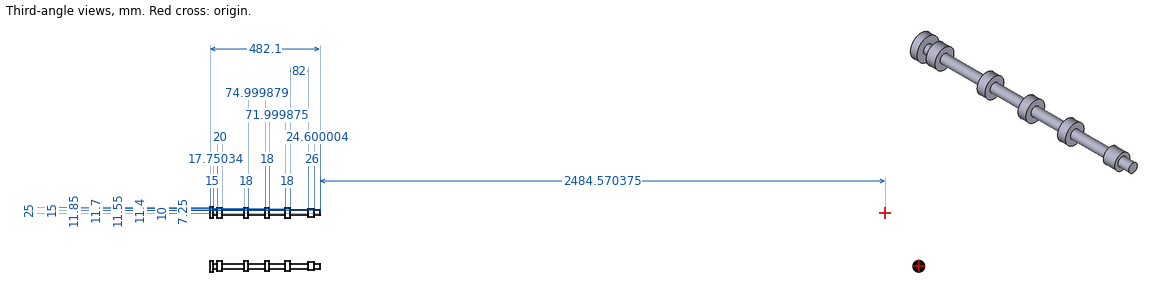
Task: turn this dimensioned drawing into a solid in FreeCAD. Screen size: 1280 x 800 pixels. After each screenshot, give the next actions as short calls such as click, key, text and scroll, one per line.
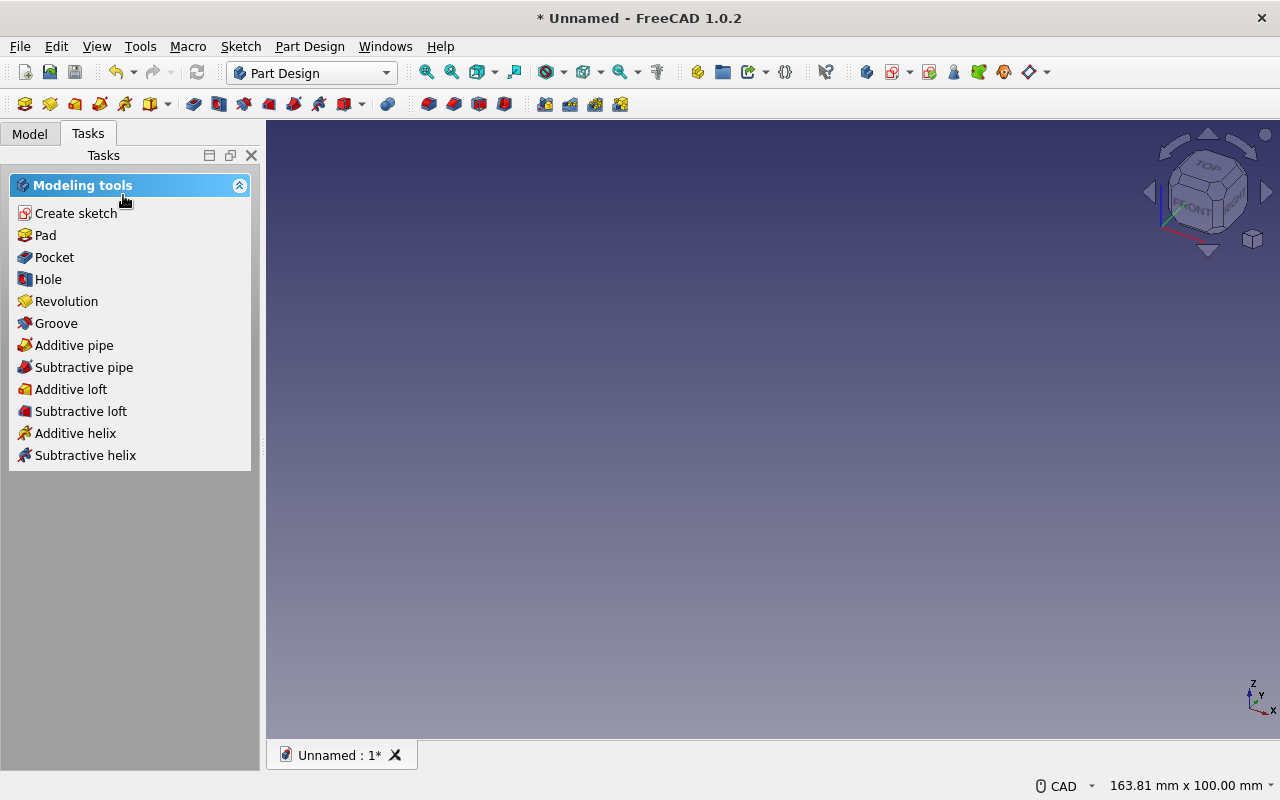
click(50, 104)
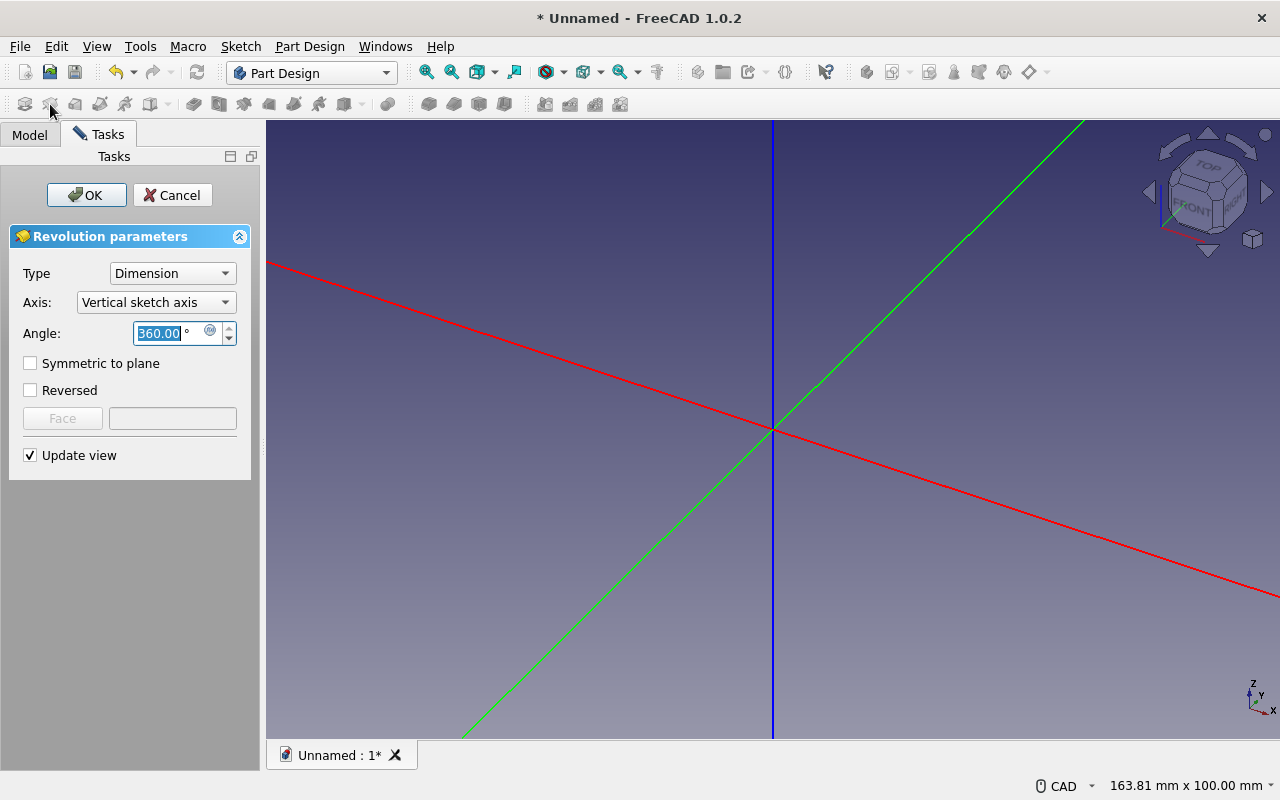
click(157, 302)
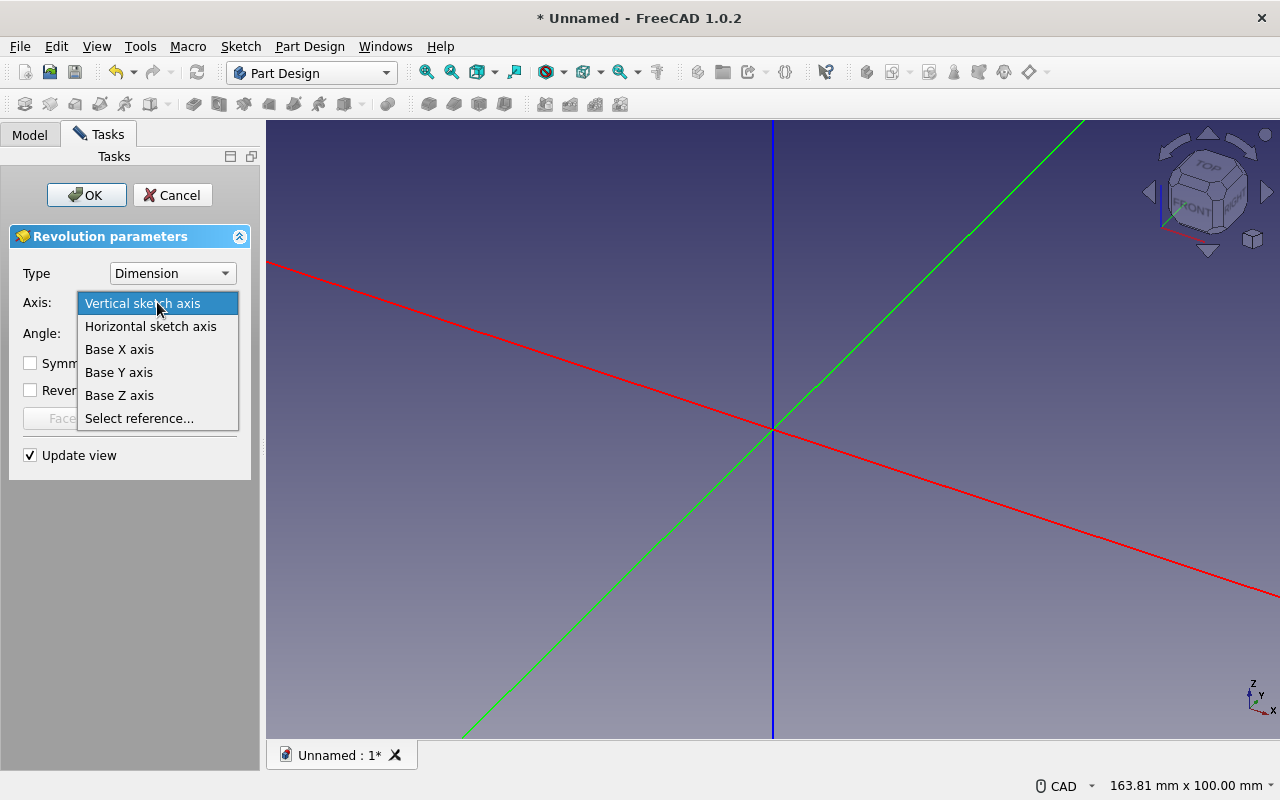
click(156, 326)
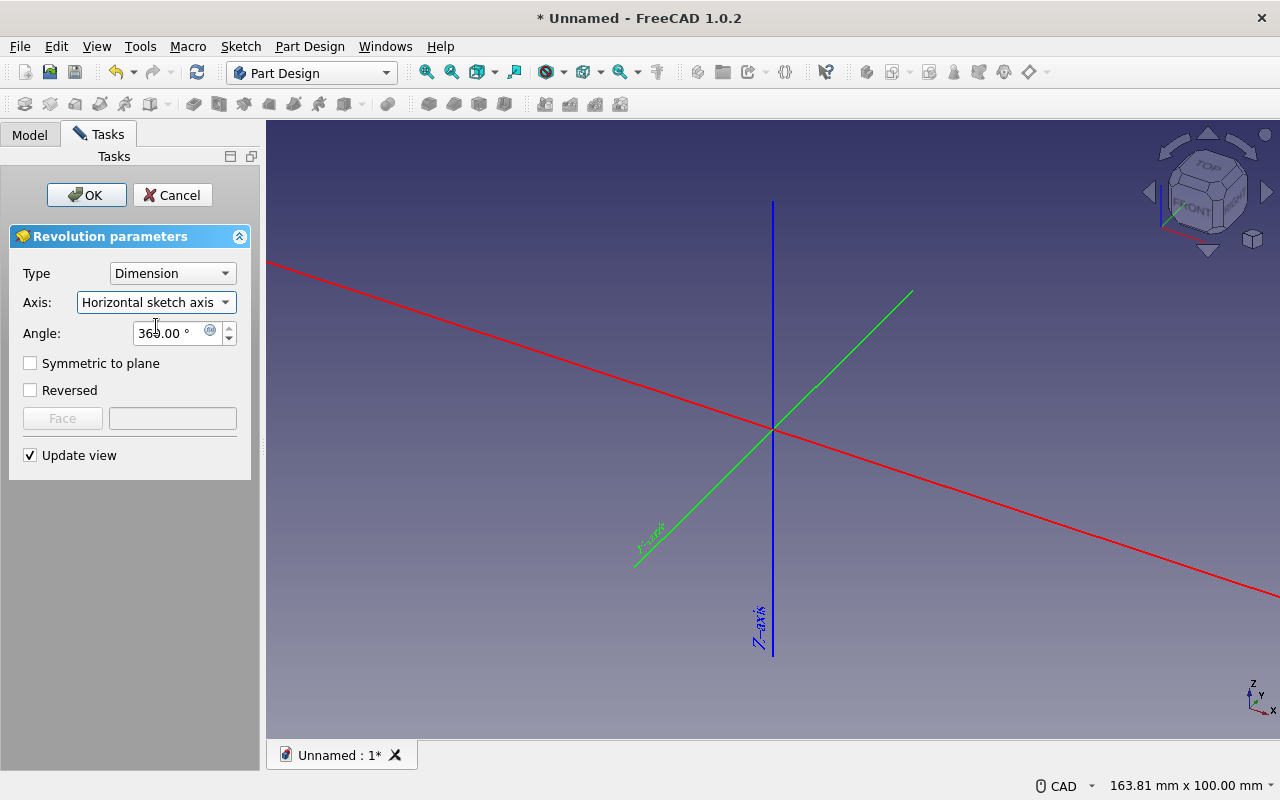
click(87, 195)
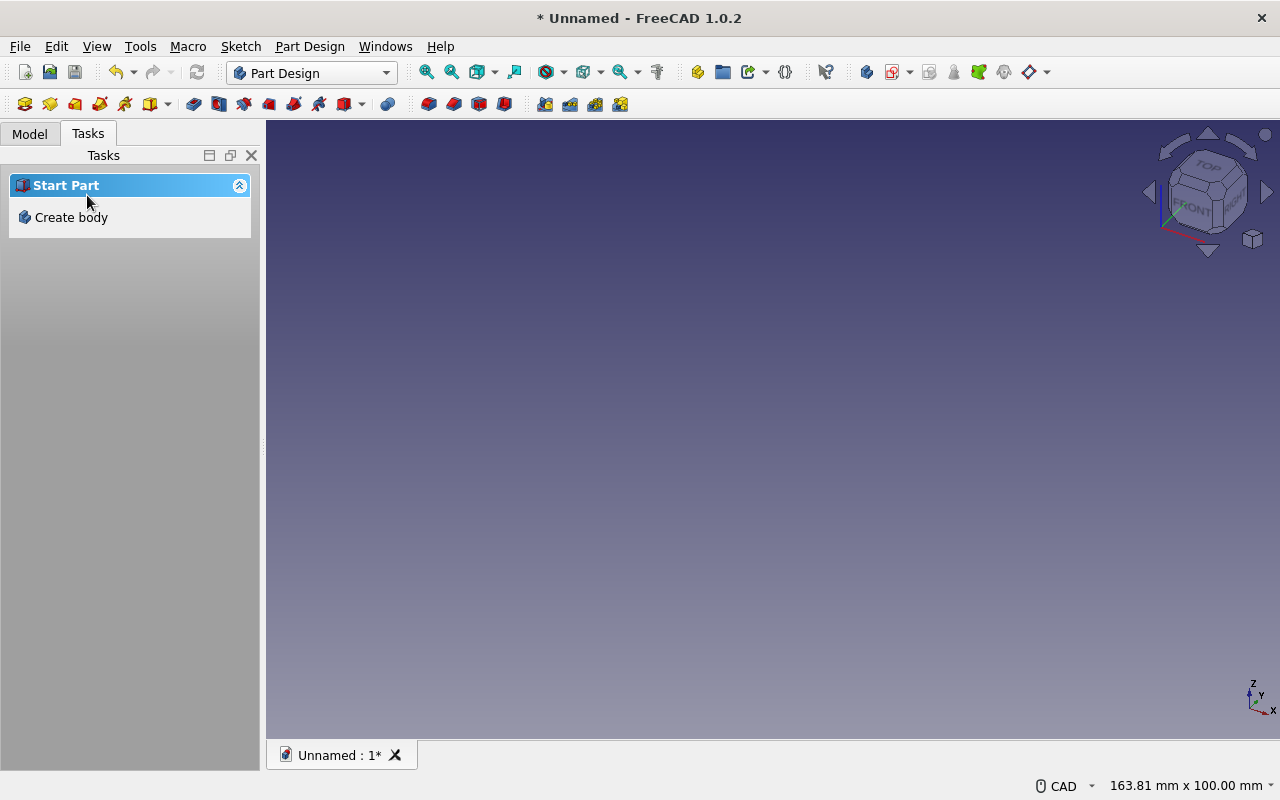
key(0)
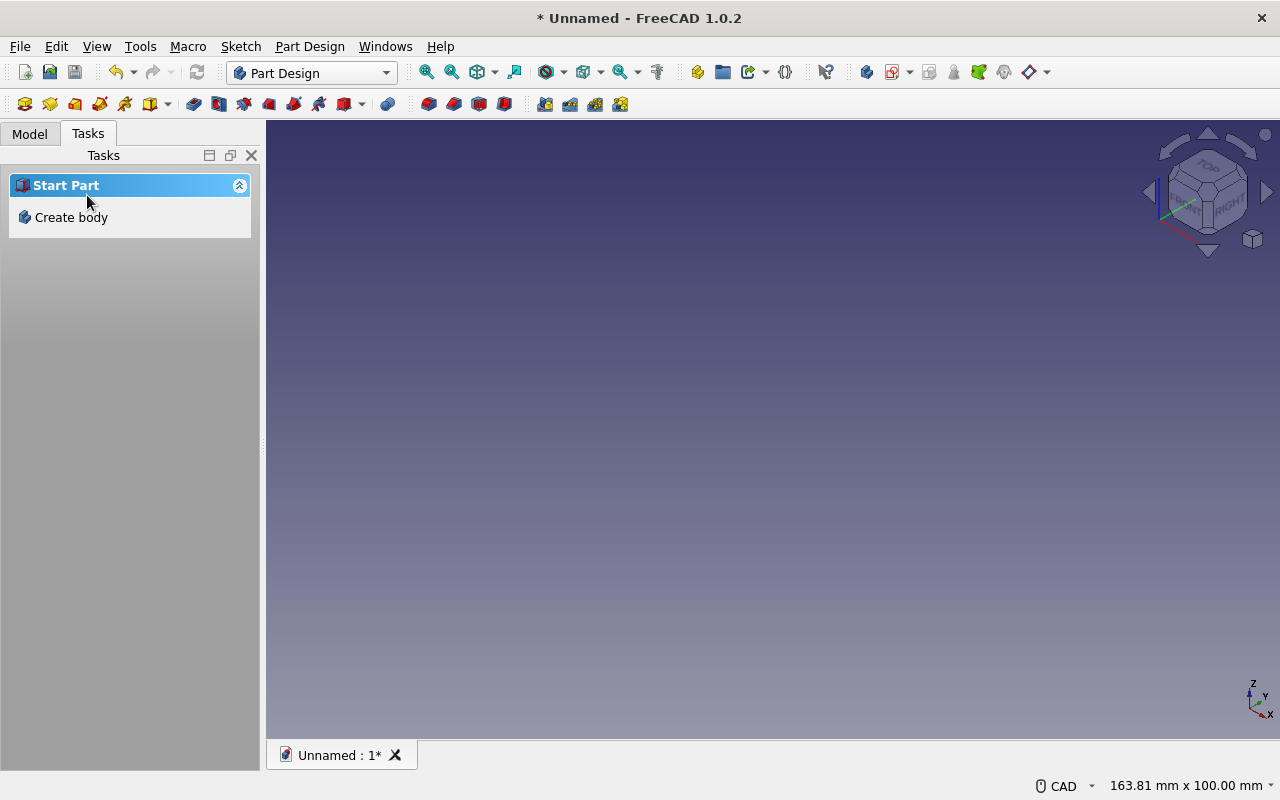
click(427, 72)